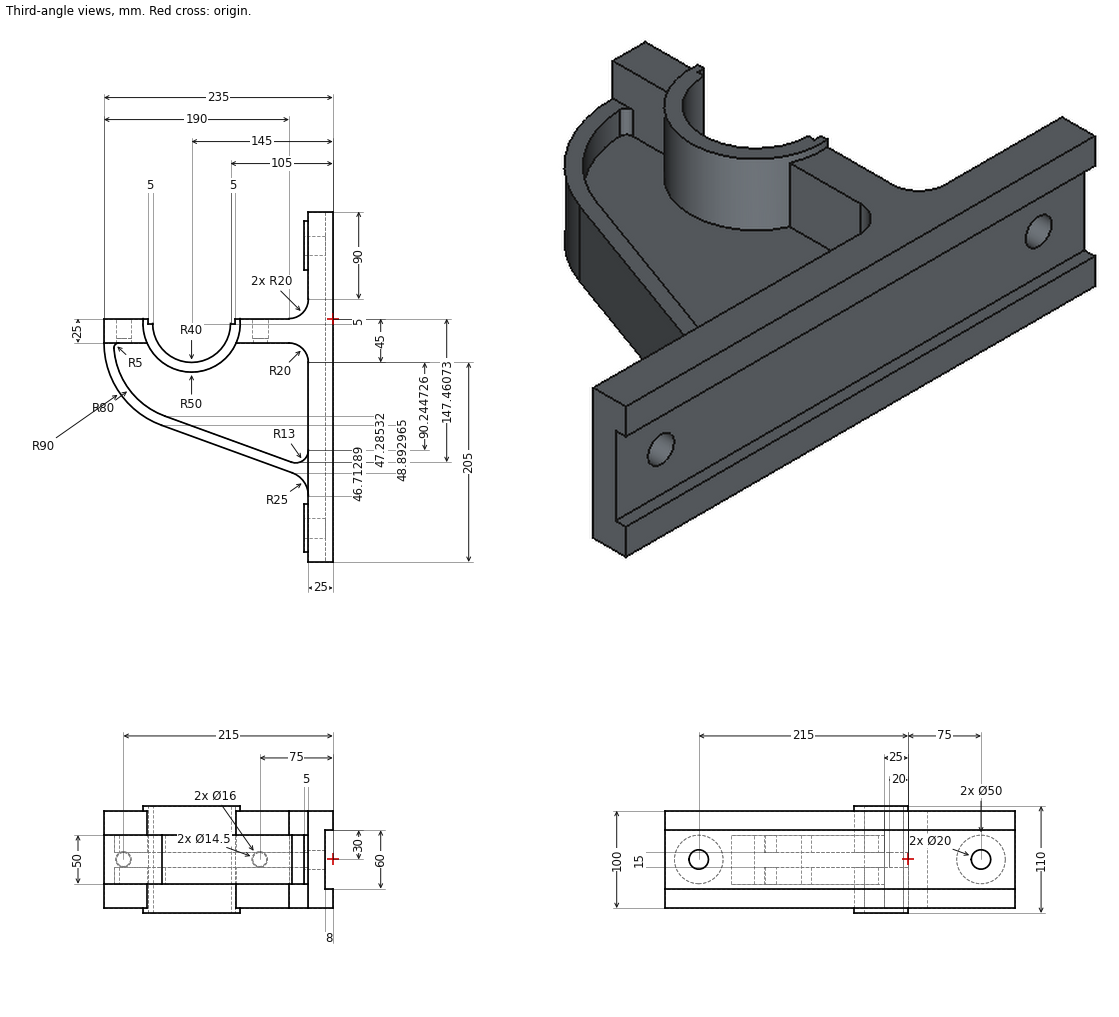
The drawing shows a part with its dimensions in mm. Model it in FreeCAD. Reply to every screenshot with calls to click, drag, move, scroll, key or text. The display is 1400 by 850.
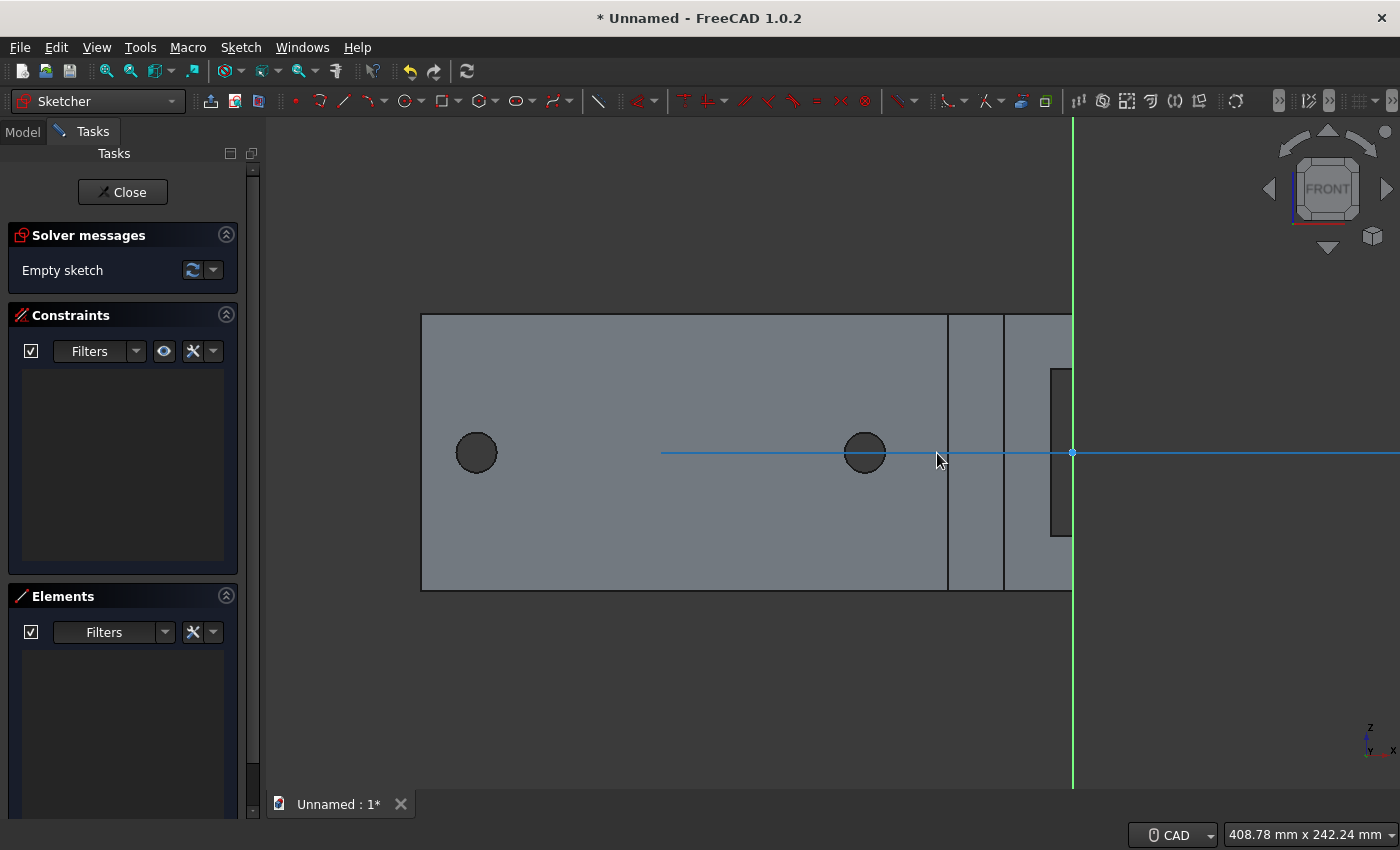
click(406, 102)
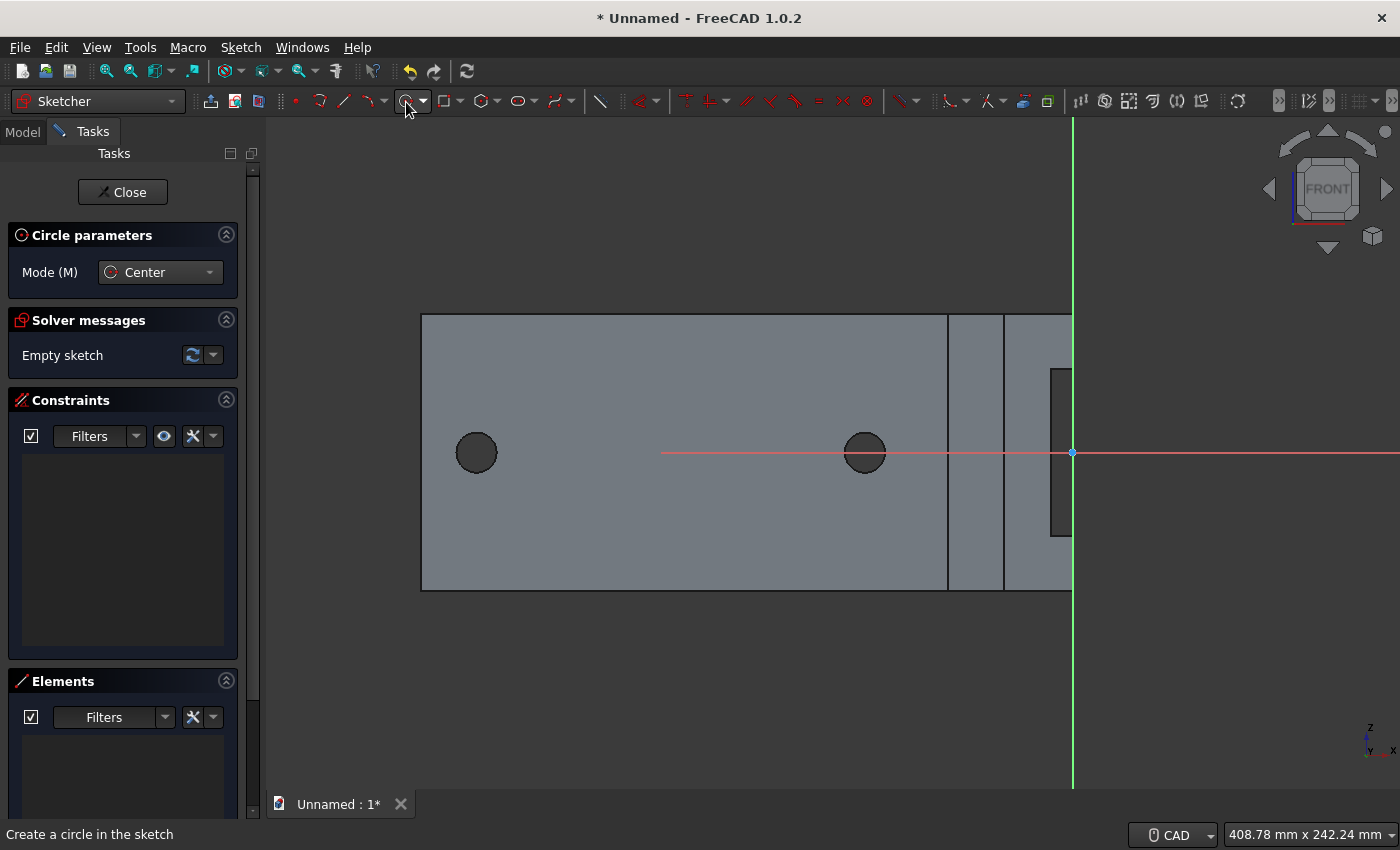
click(865, 453)
move(881, 437)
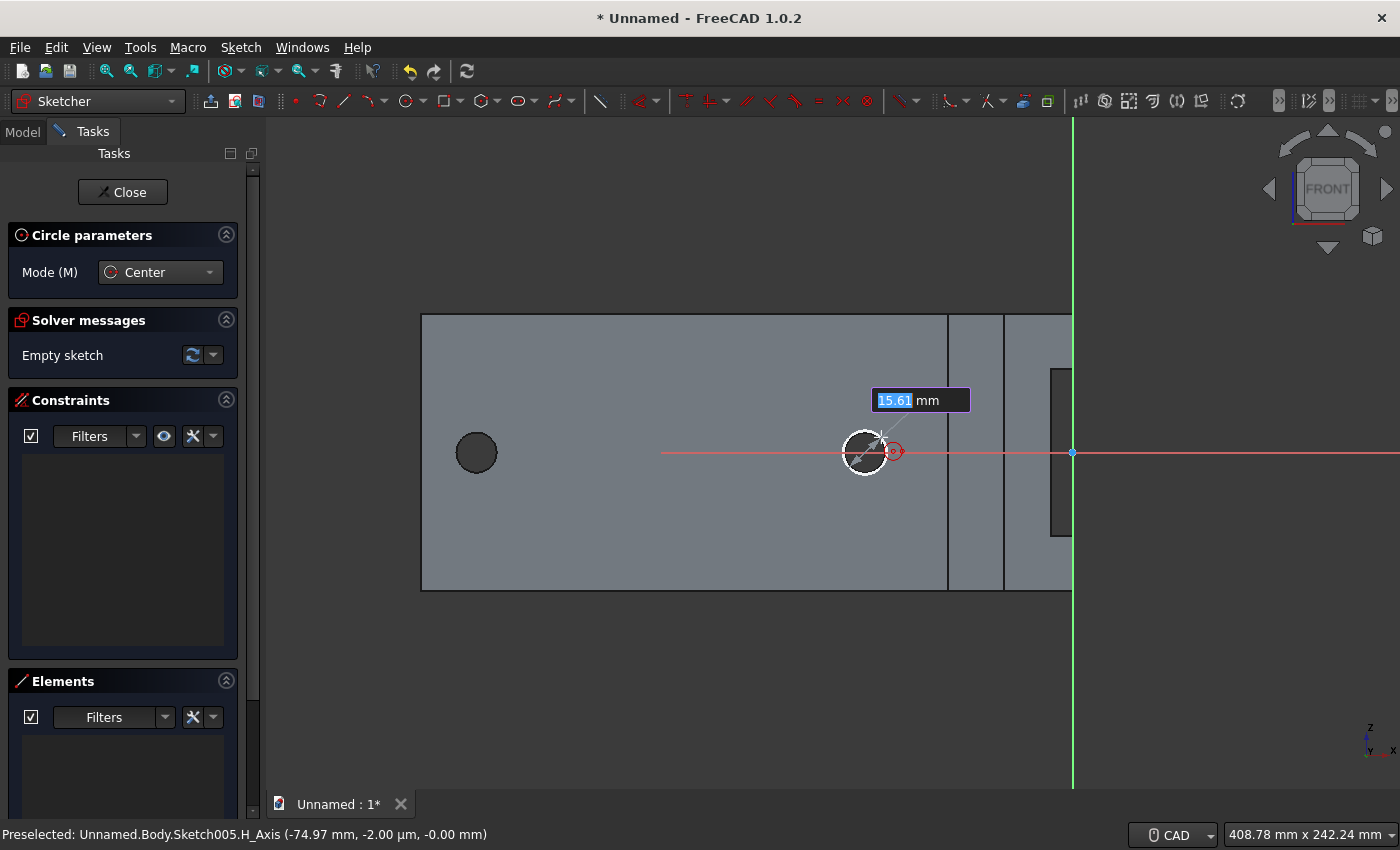
text(16)
key(Return)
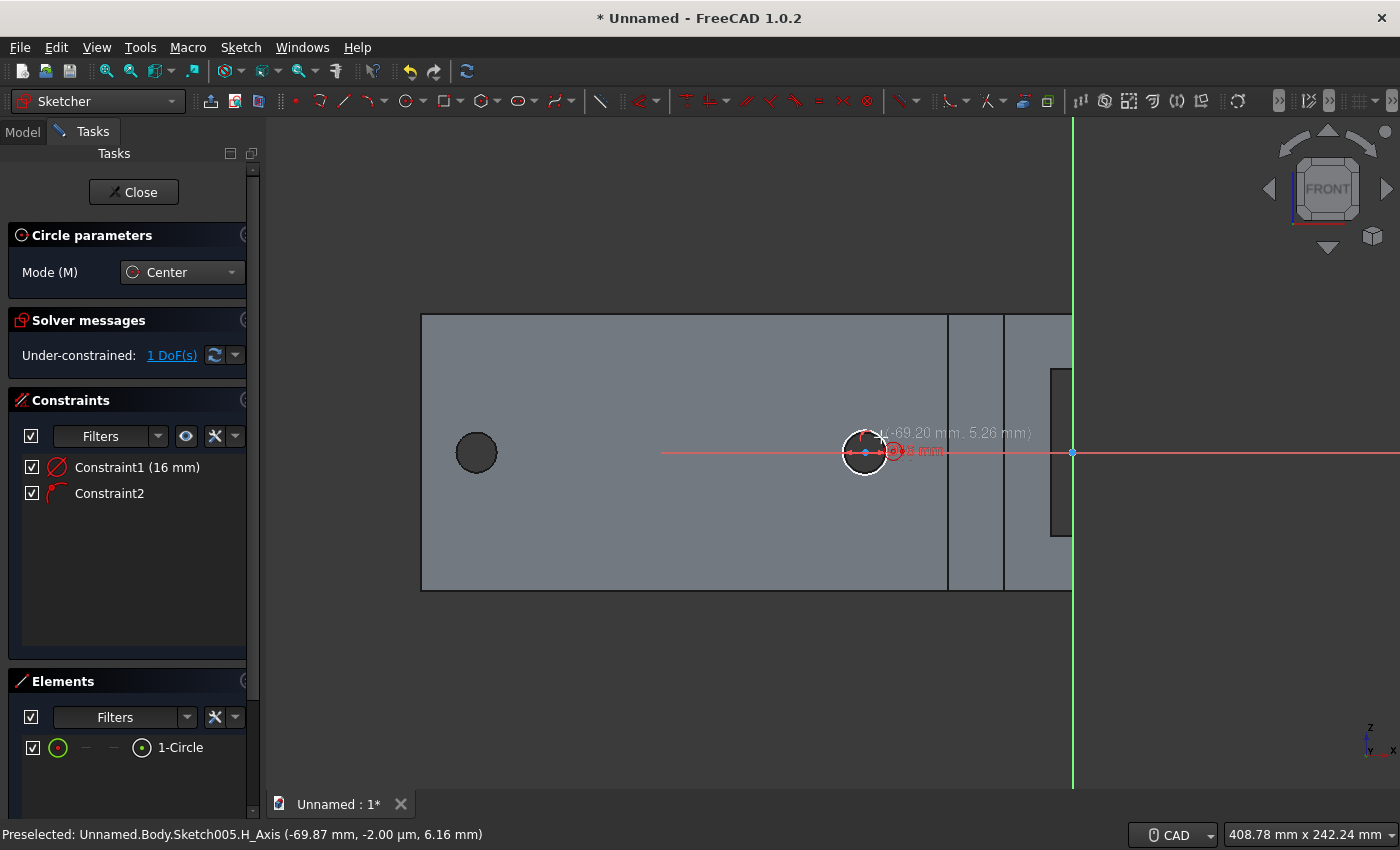
click(477, 453)
move(492, 437)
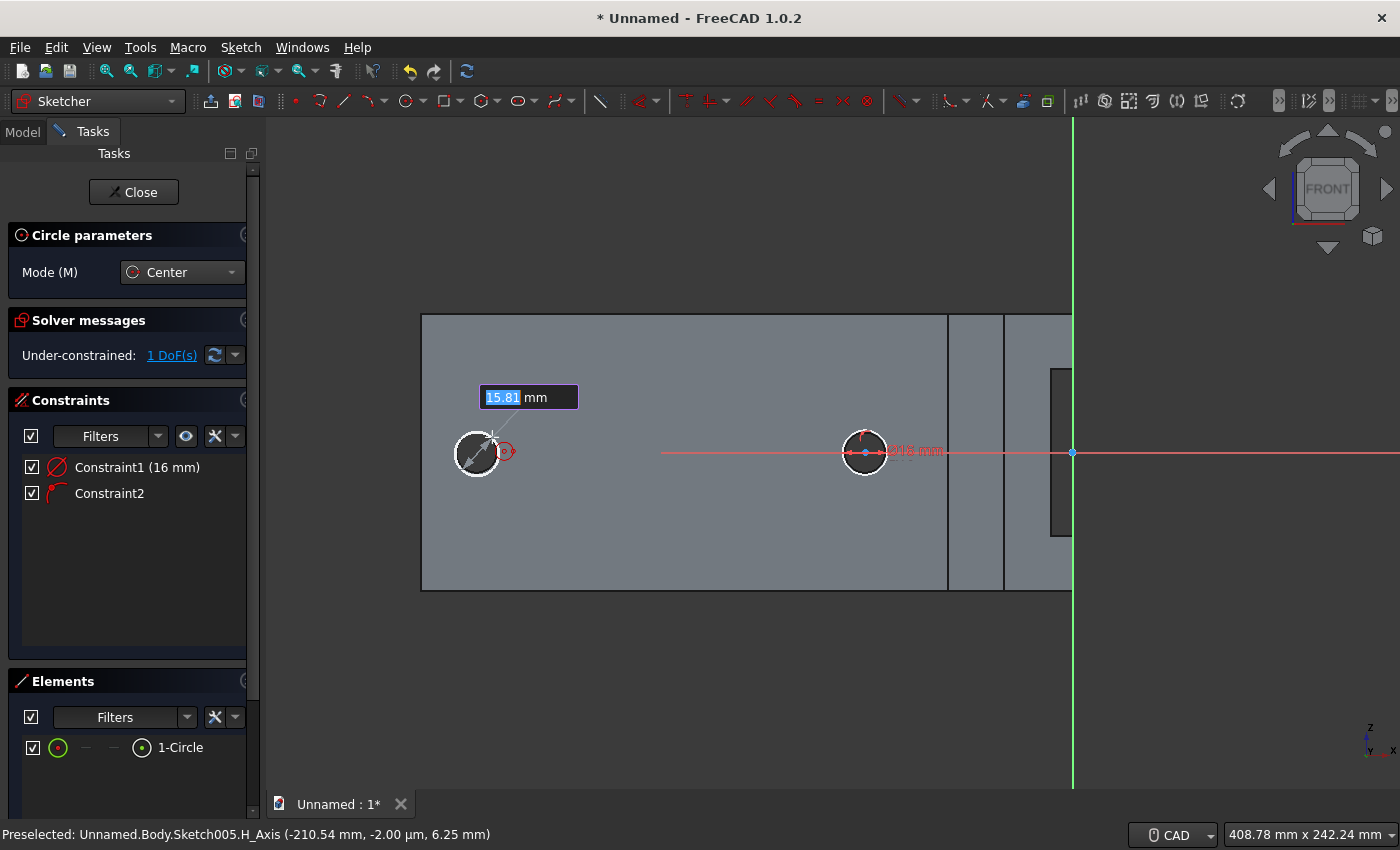
text(16)
key(Return)
key(Escape)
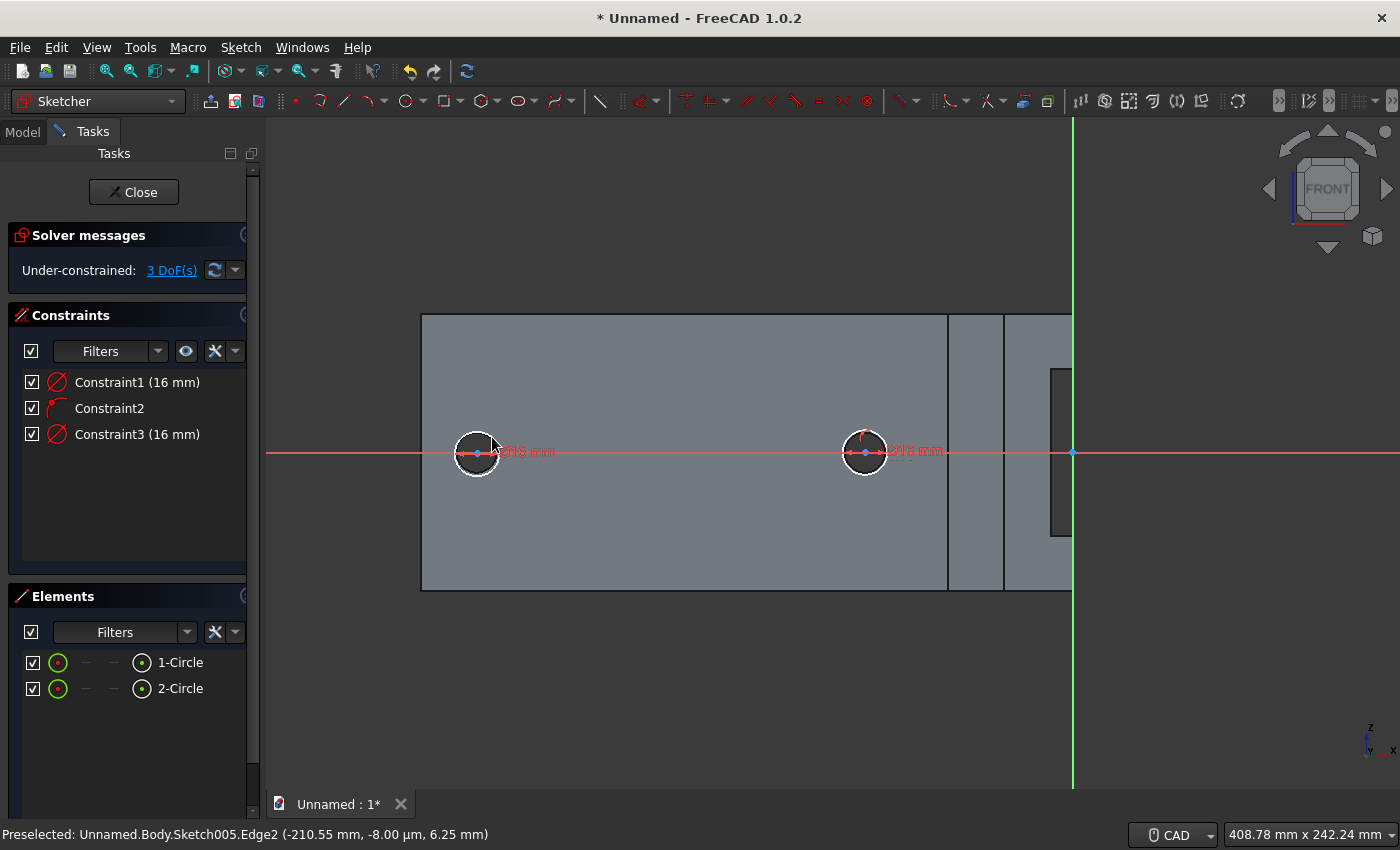
click(477, 454)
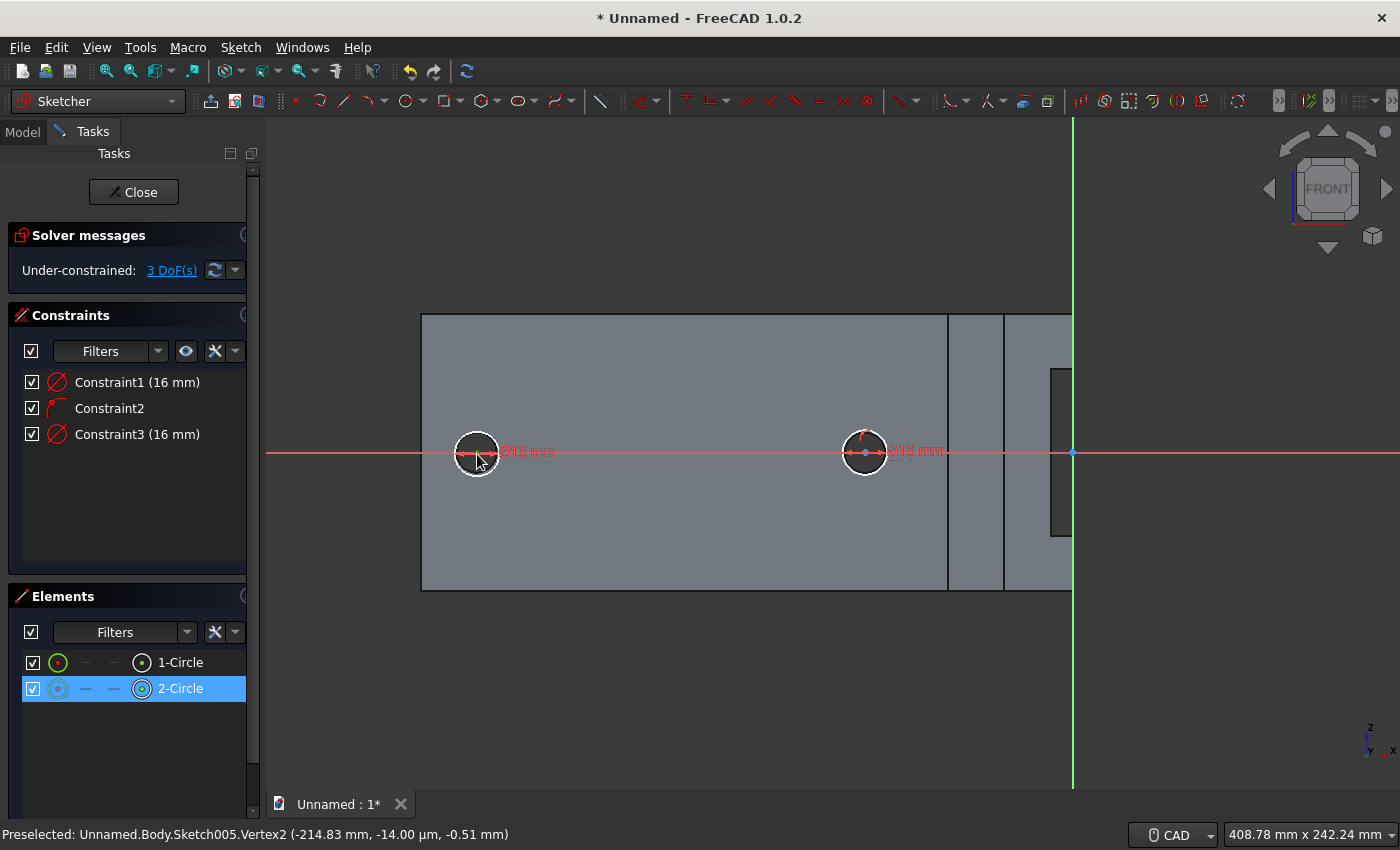
click(361, 453)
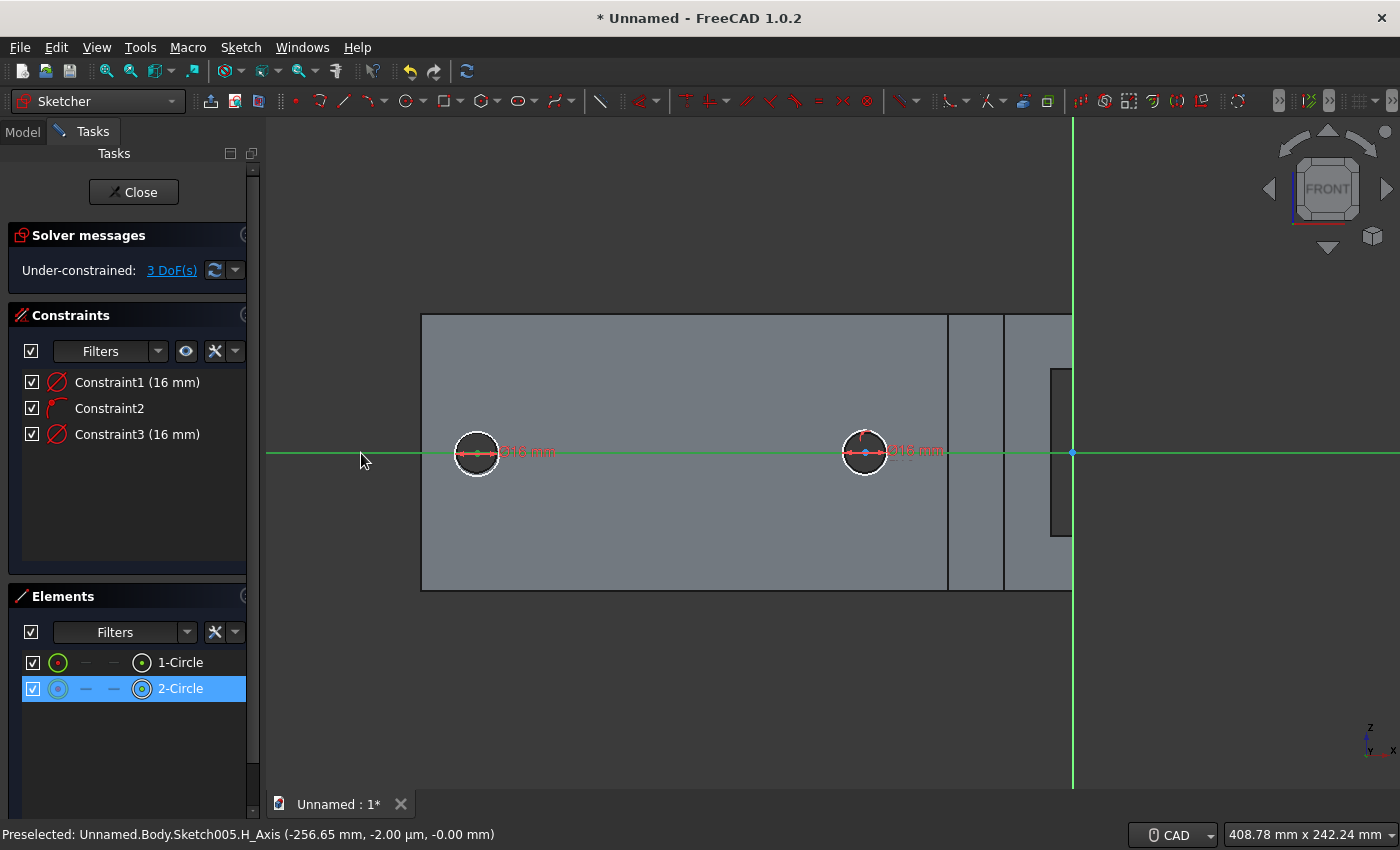
click(686, 102)